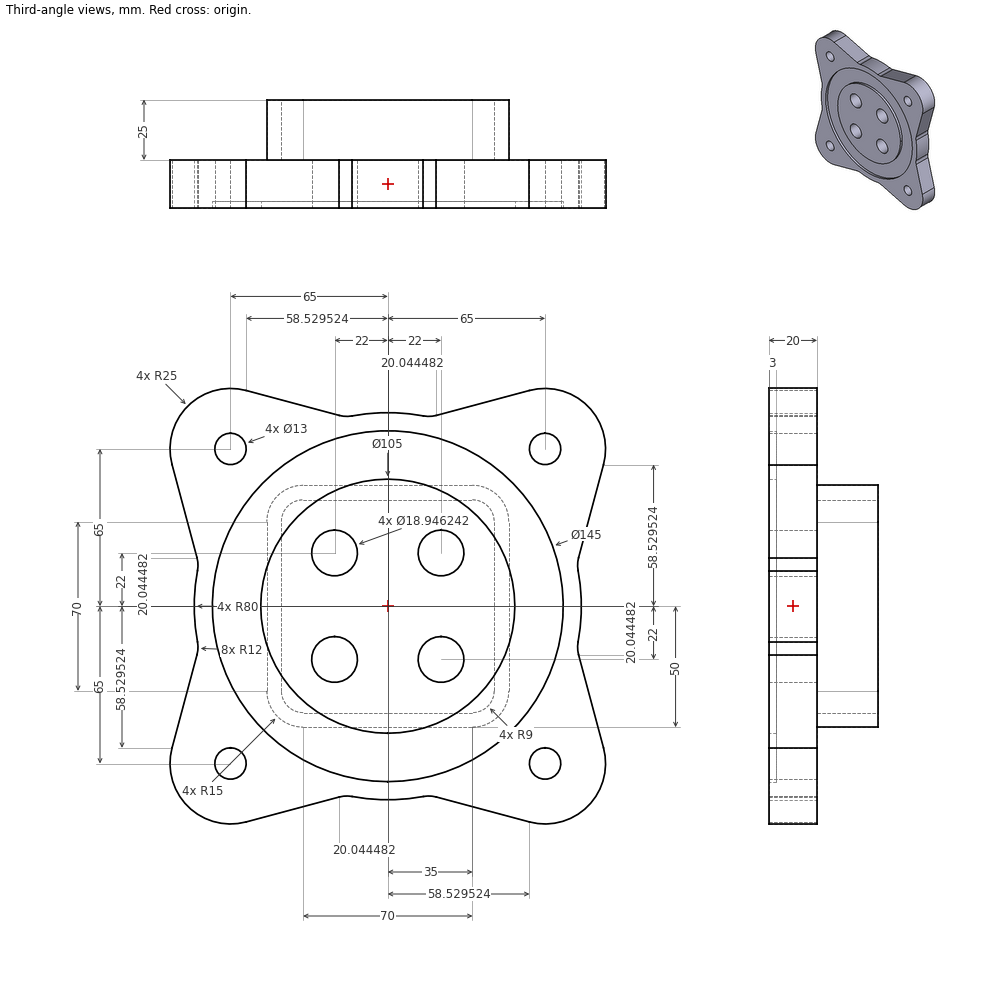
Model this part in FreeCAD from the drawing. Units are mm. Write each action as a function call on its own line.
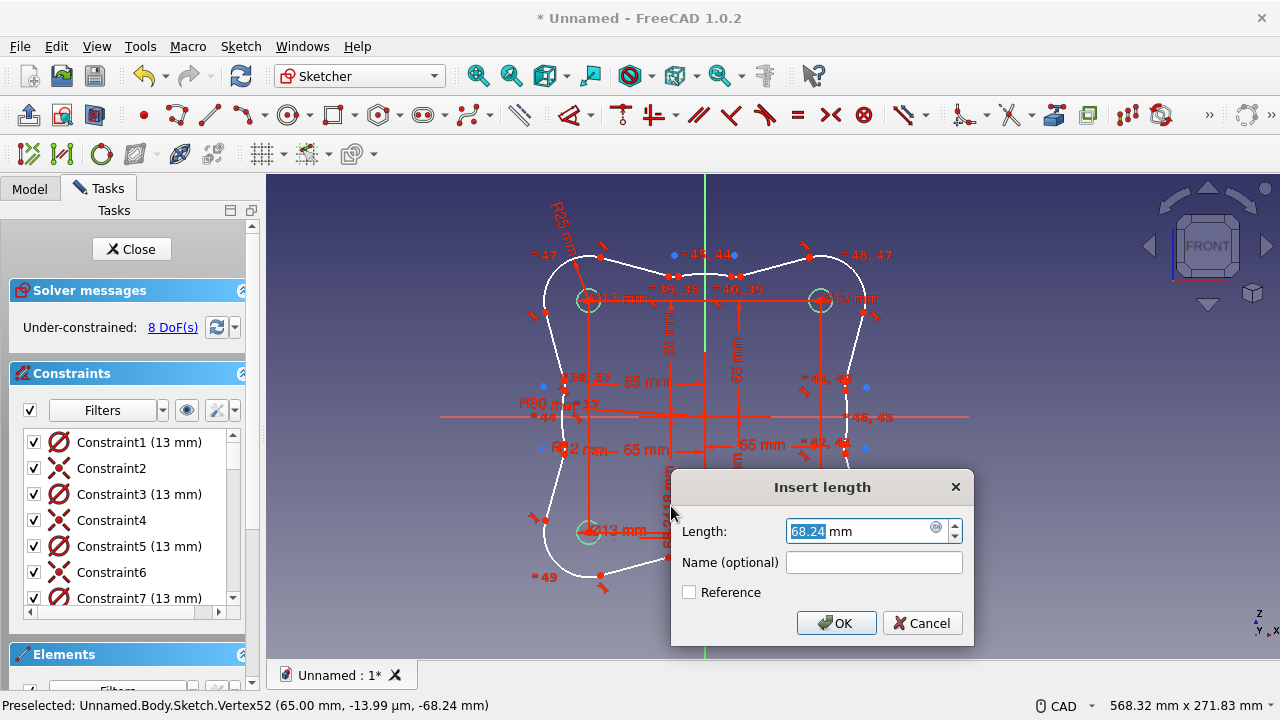
text(65)
key(Return)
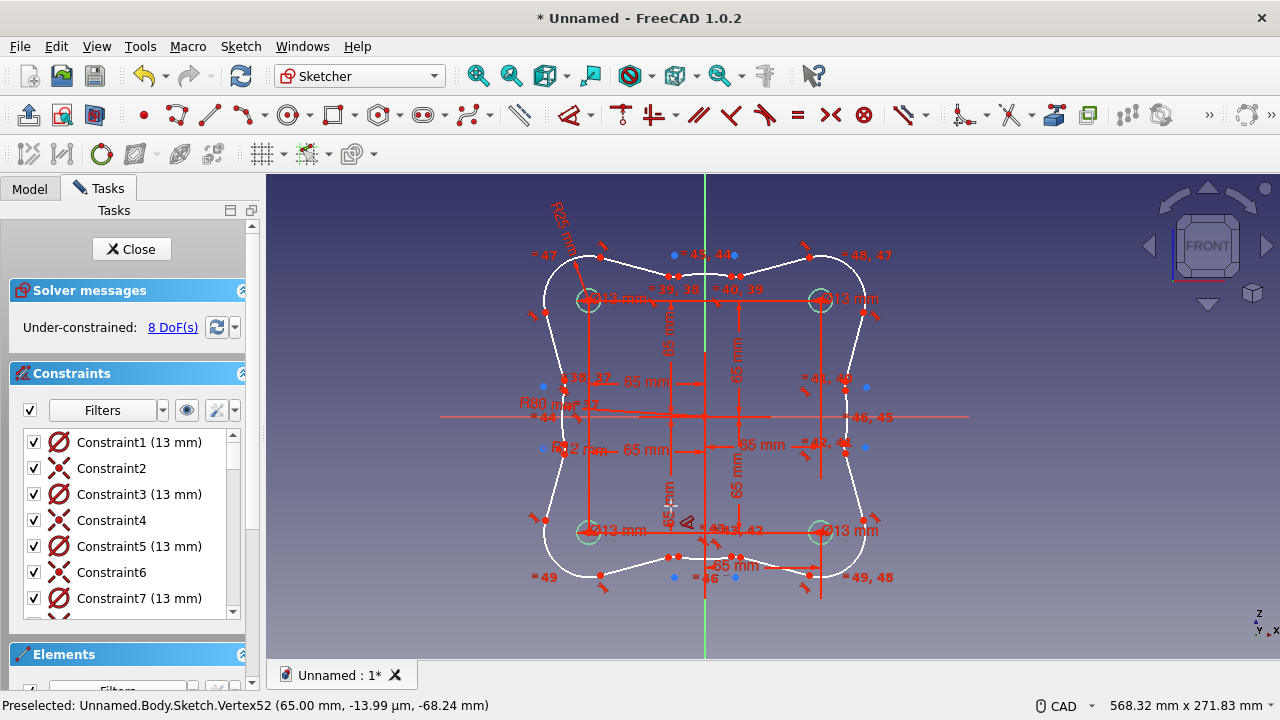
click(546, 521)
click(512, 469)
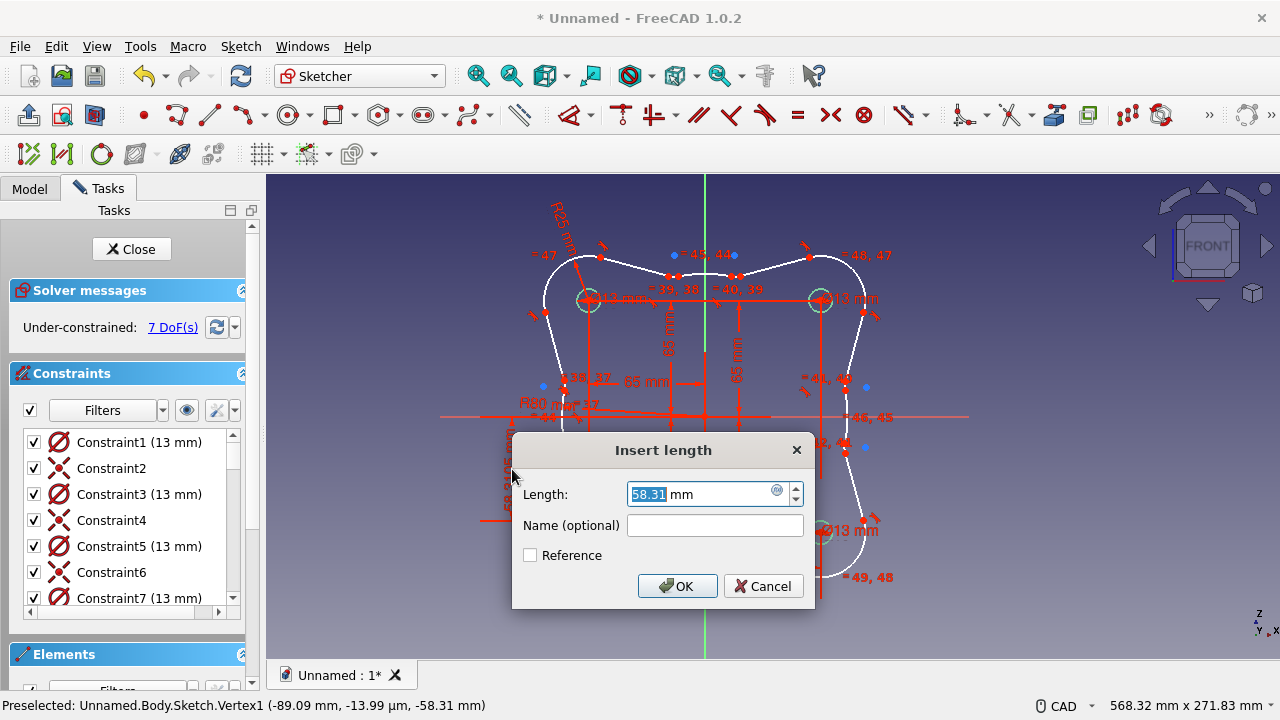
text(58.529524)
key(Return)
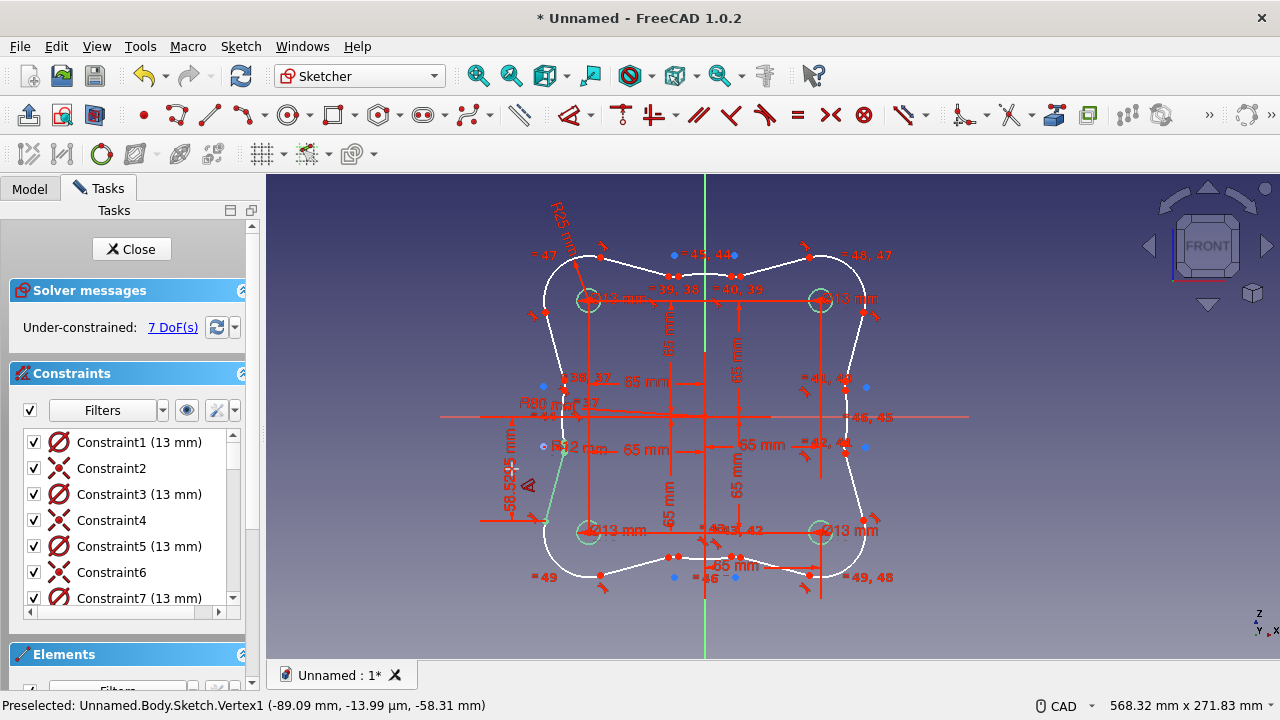
scroll(564, 381, up, 2)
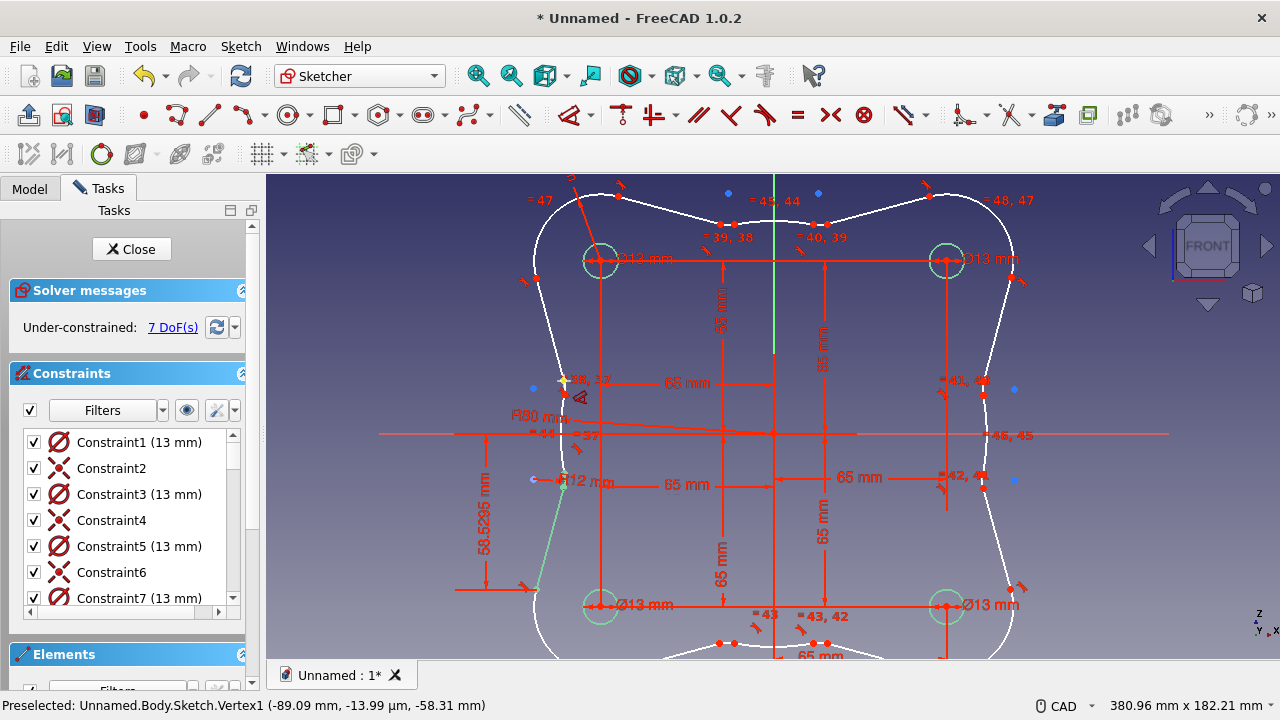
click(564, 381)
click(530, 395)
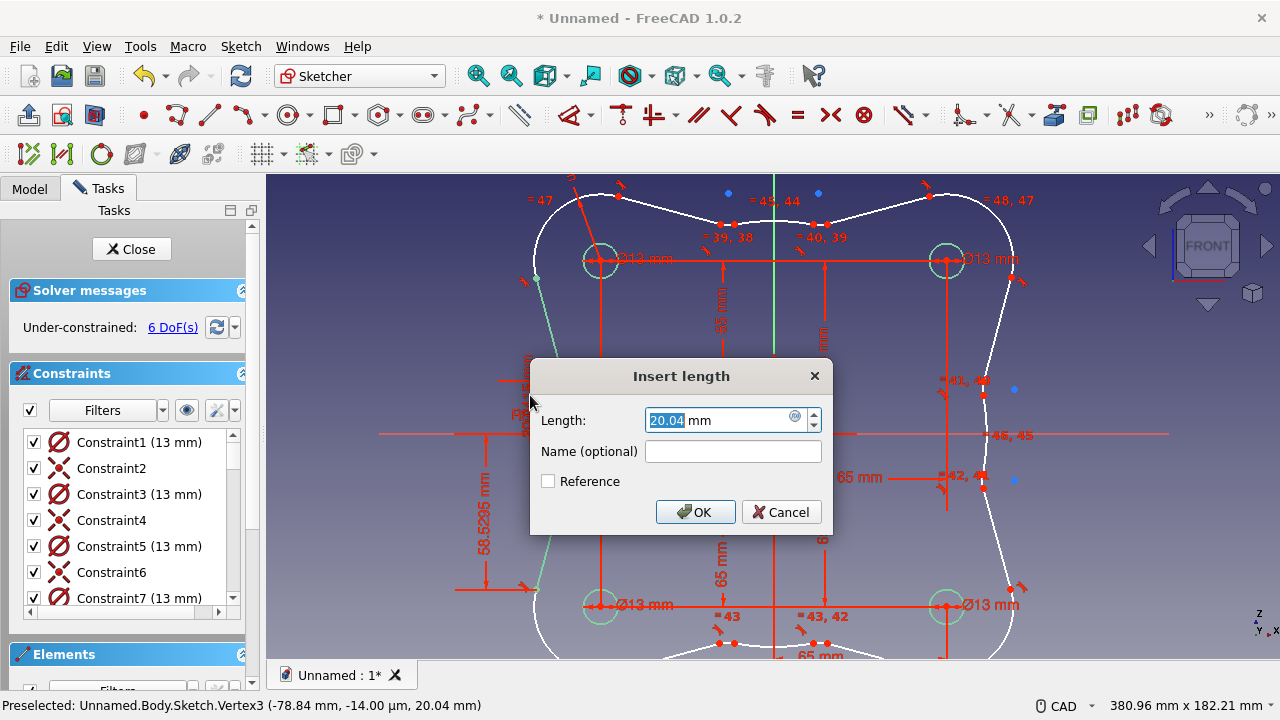
text(20.044482)
key(Return)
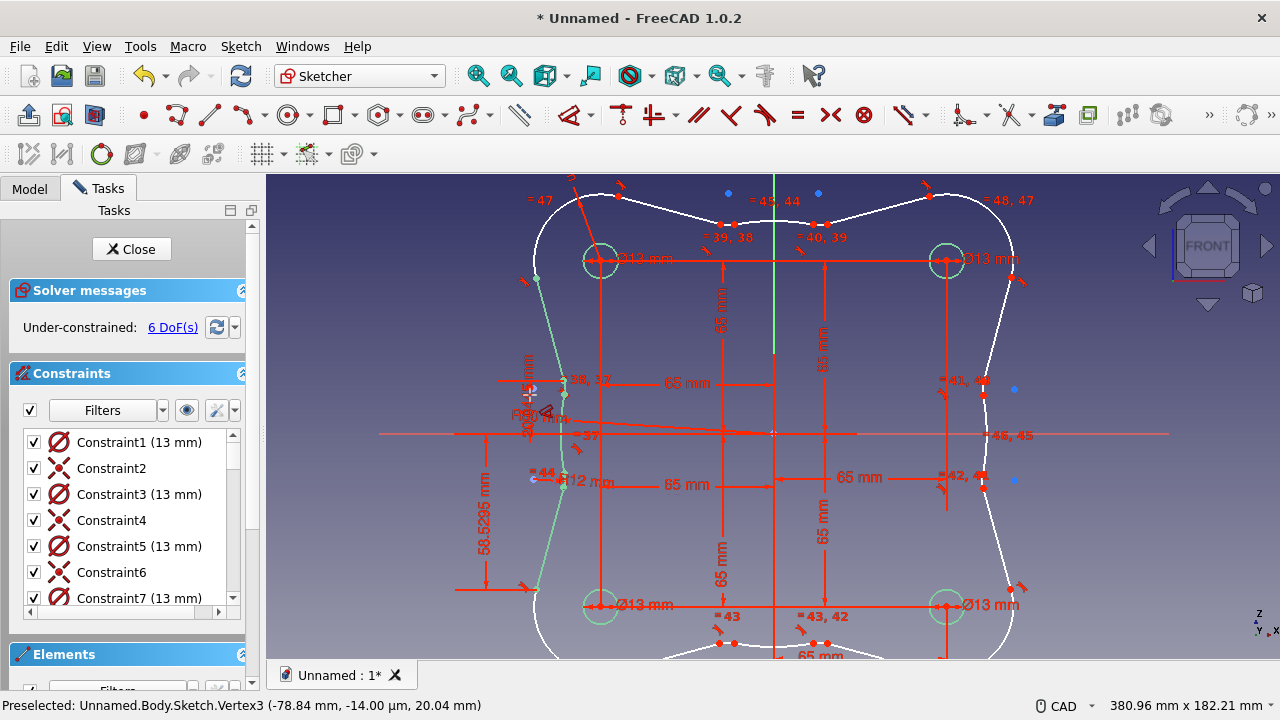
scroll(564, 381, down, 2)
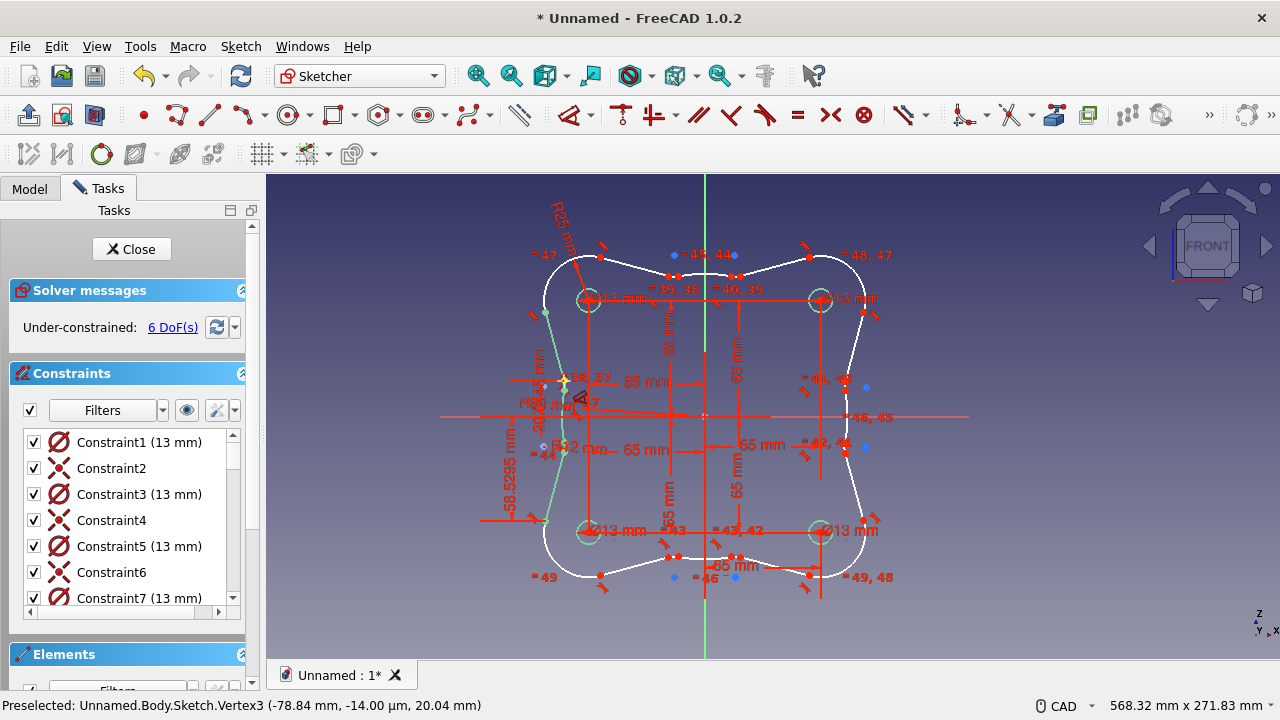
click(600, 258)
click(652, 224)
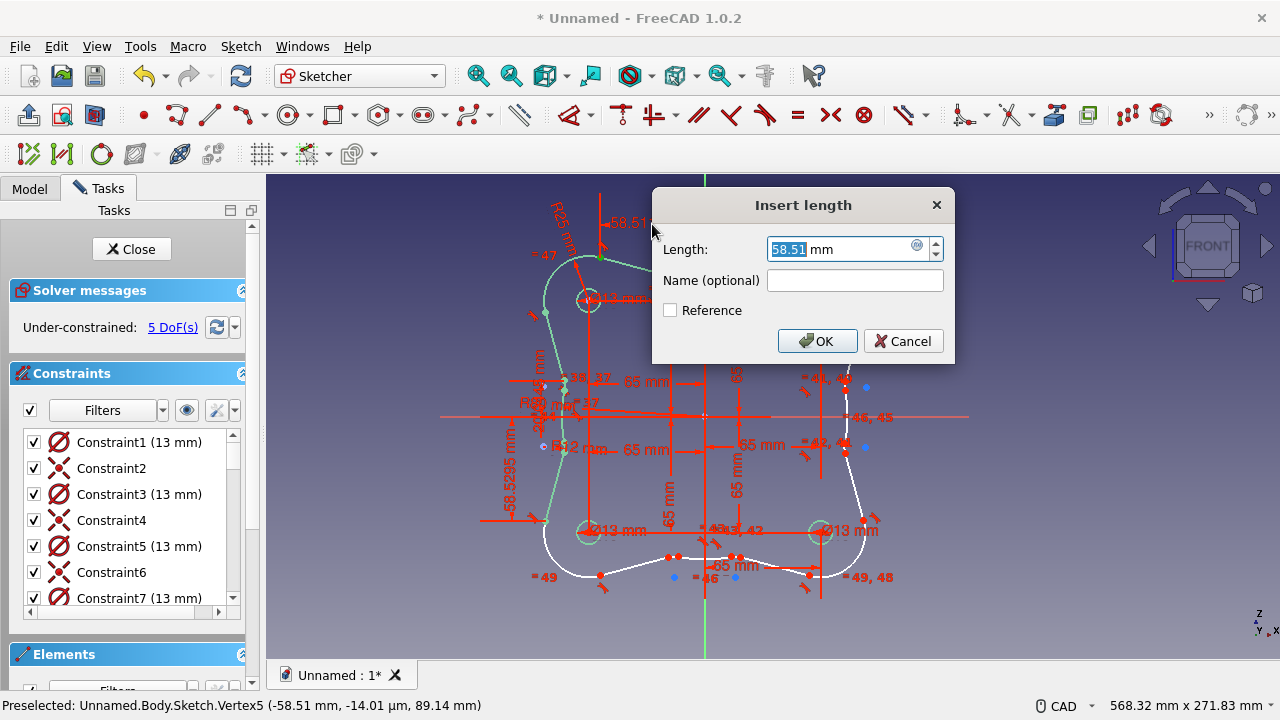
text(58.529524)
key(Return)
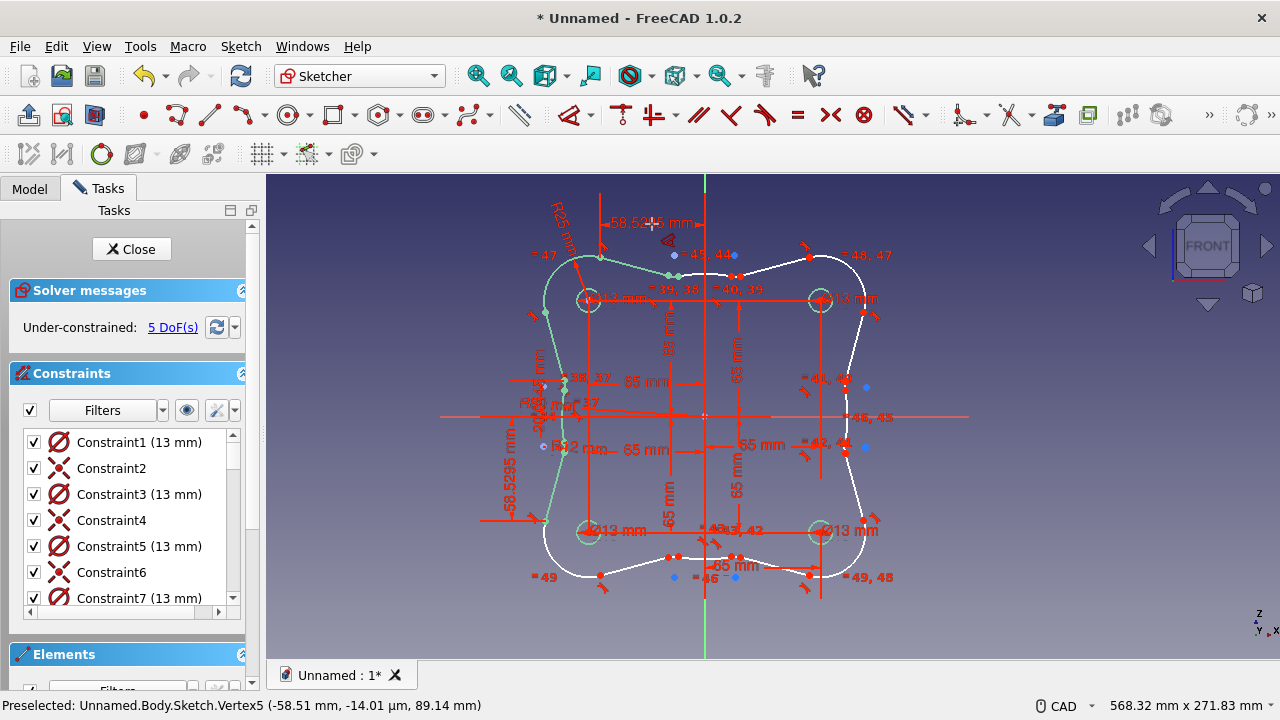
scroll(741, 276, up, 2)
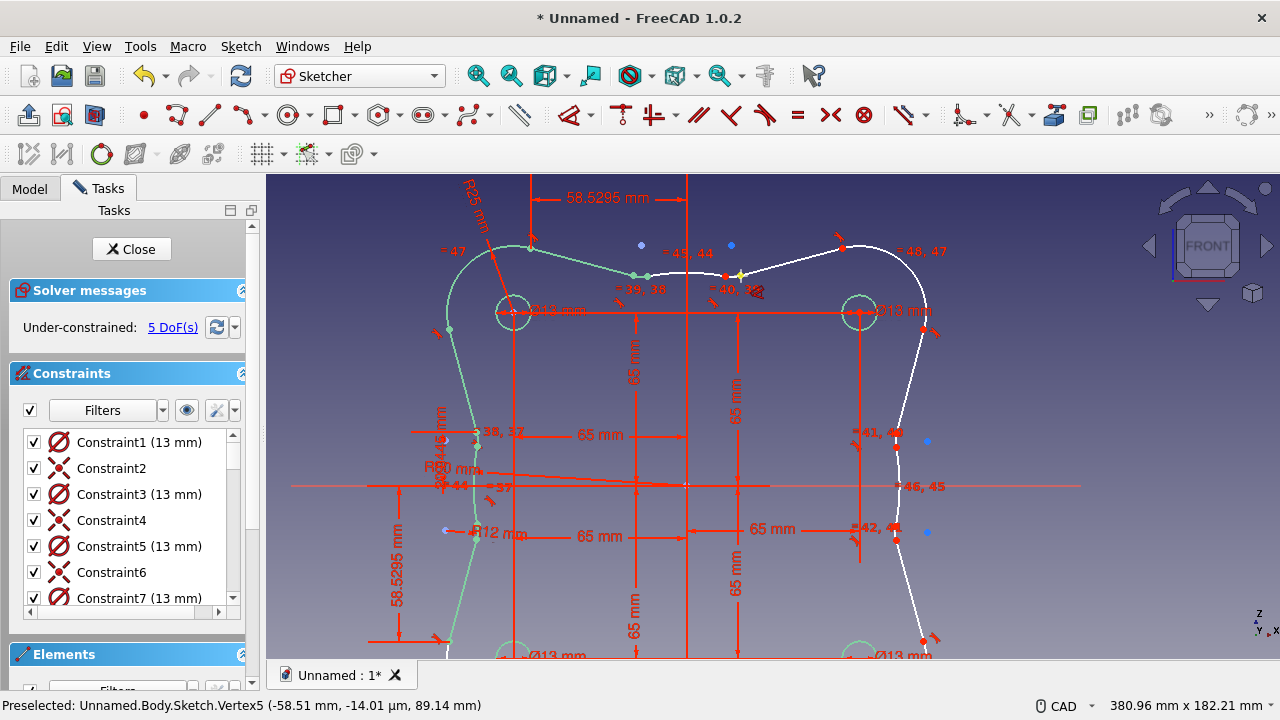
click(740, 276)
click(713, 242)